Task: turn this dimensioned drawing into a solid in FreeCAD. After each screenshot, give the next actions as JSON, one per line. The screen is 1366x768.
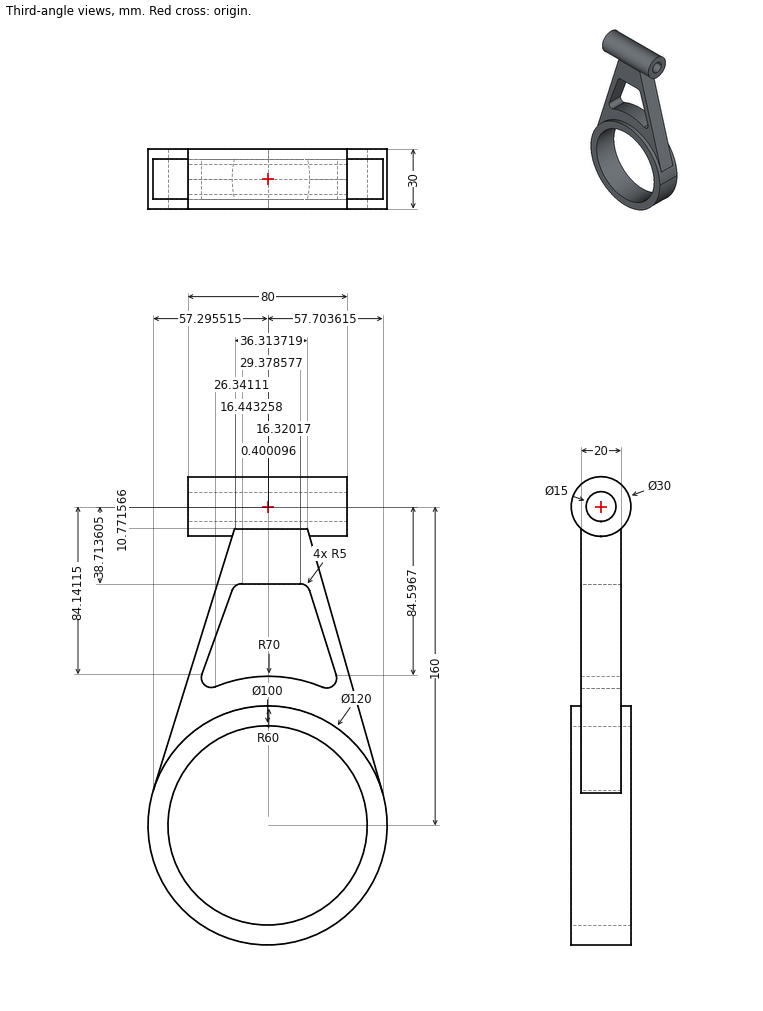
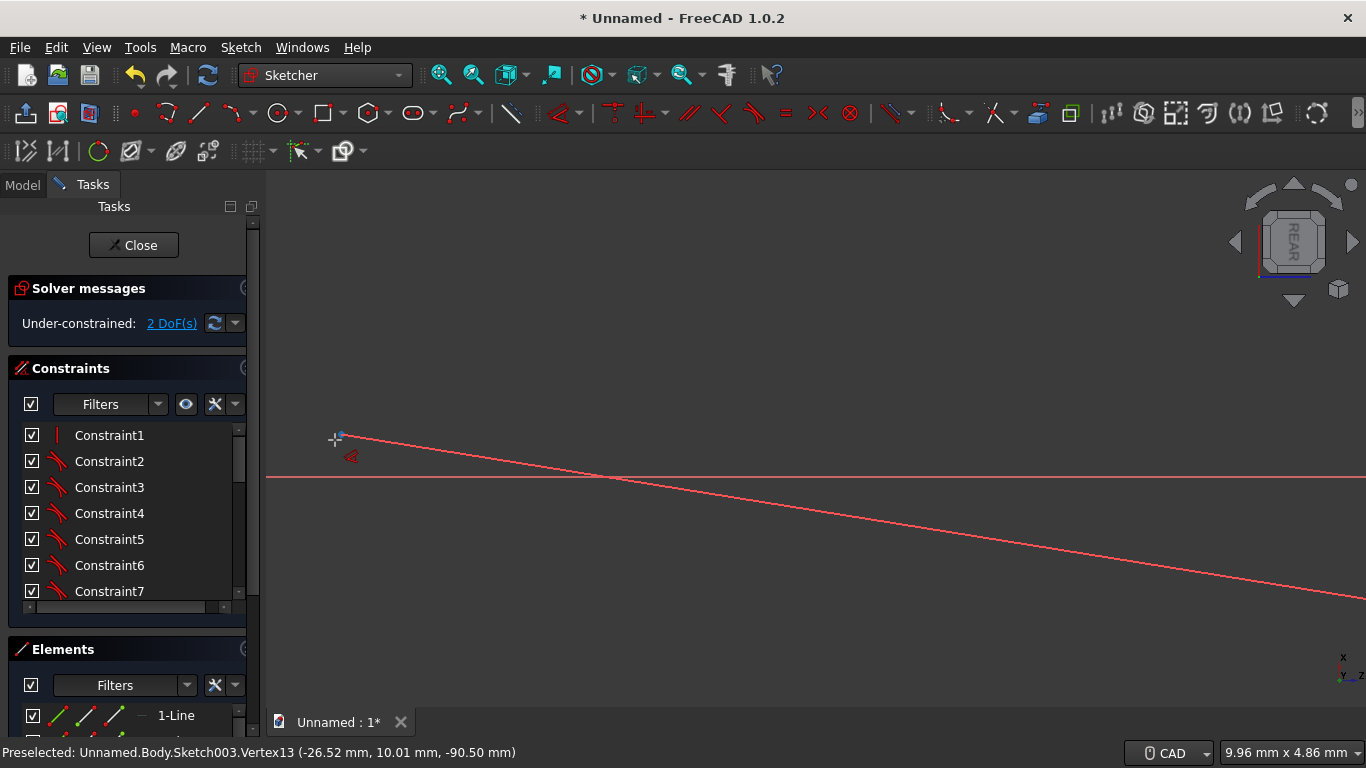
{"action": "left_click", "coordinate": [341, 435]}
{"action": "left_click", "coordinate": [307, 456]}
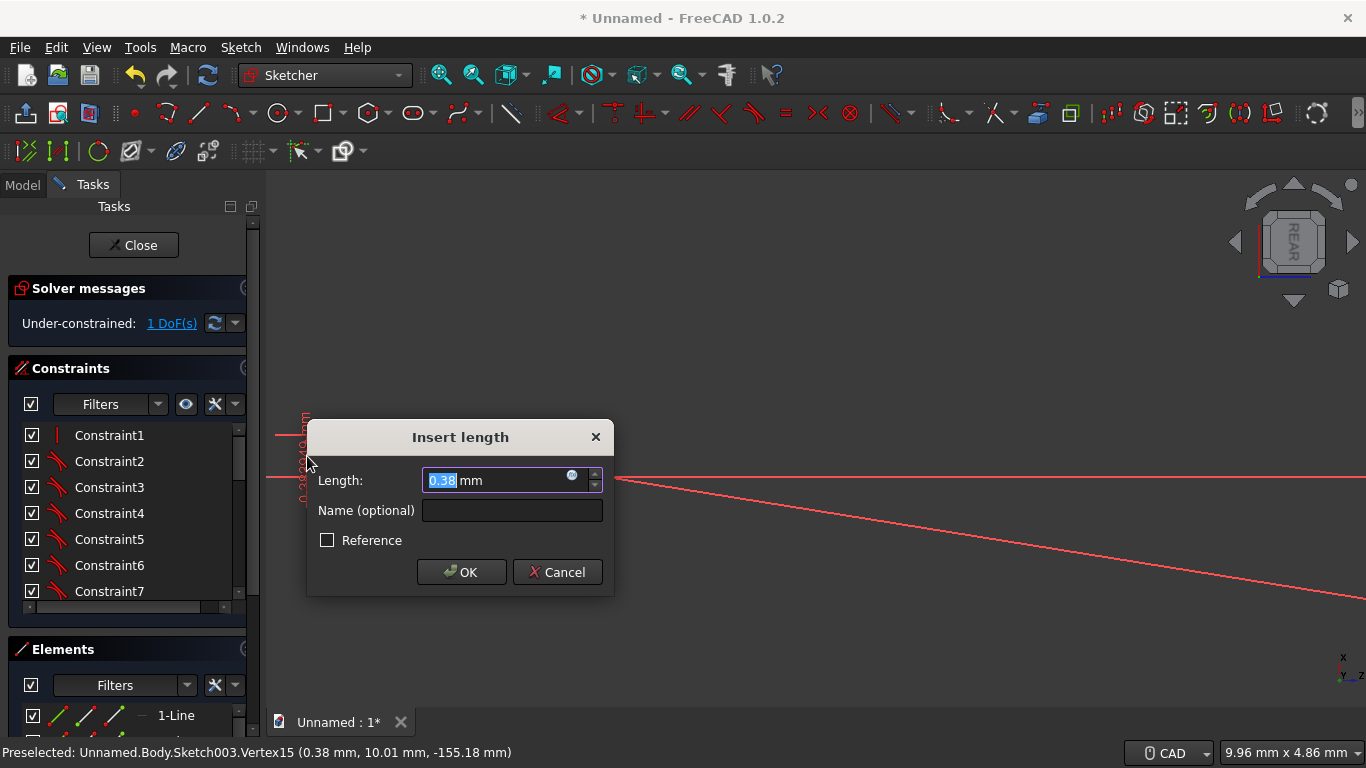
{"action": "type", "text": "0.400096"}
{"action": "key", "text": "Return"}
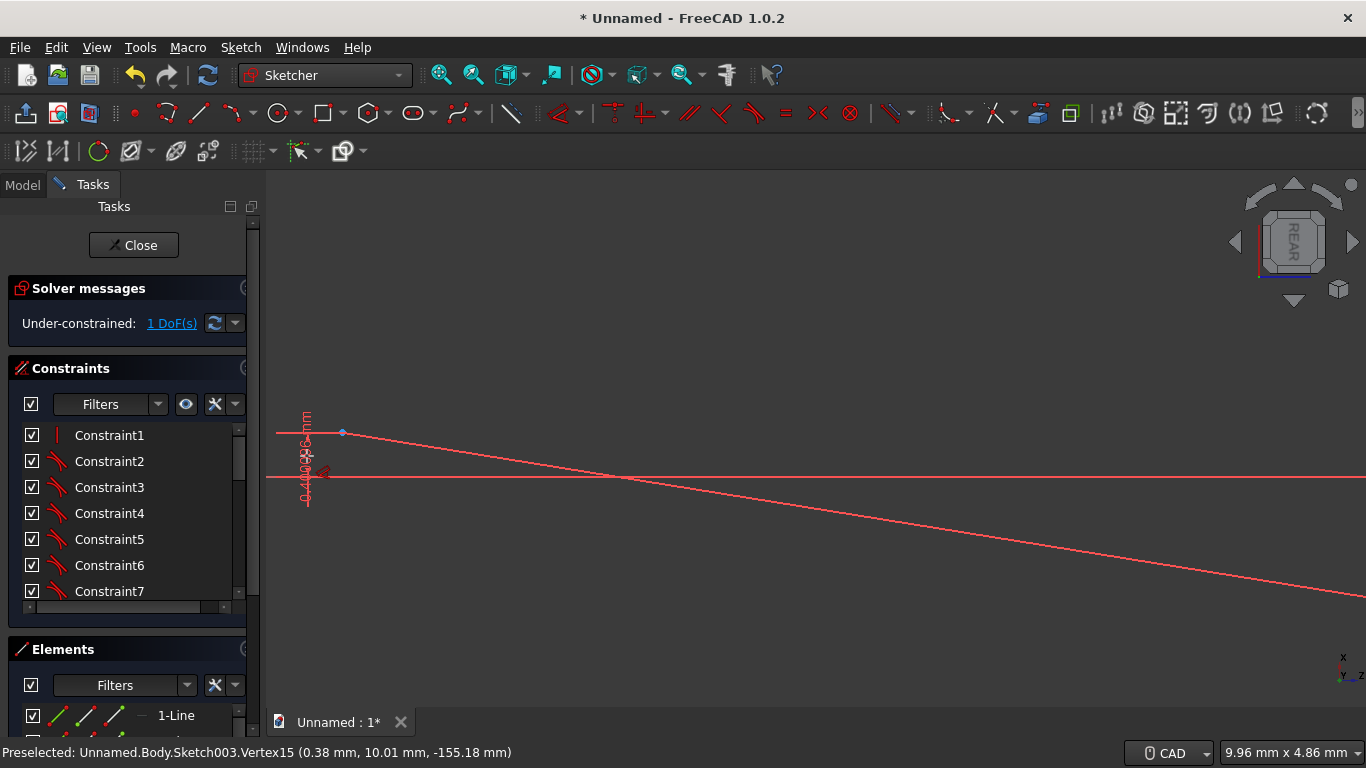
{"action": "scroll", "coordinate": [294, 441], "scroll_direction": "down", "scroll_amount": 15}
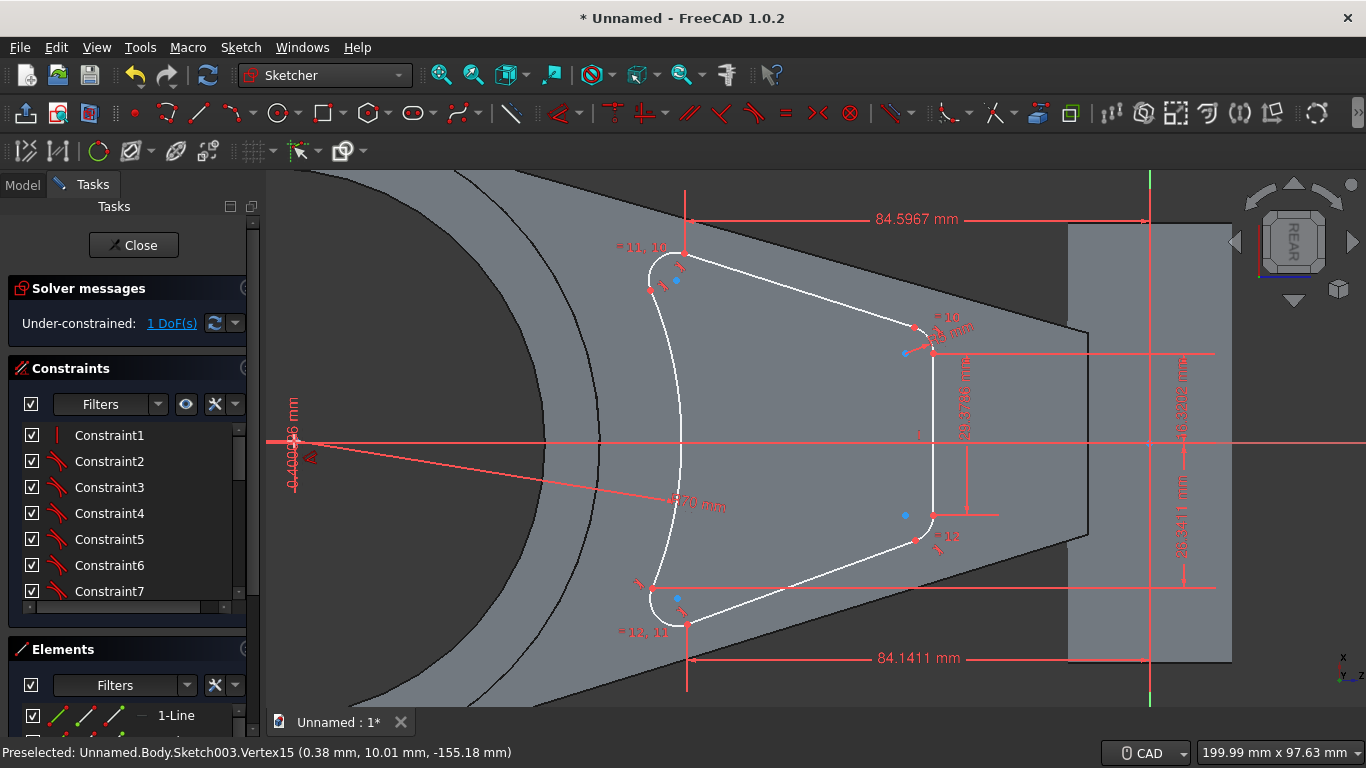
{"action": "left_click", "coordinate": [933, 515]}
{"action": "left_click", "coordinate": [1042, 549]}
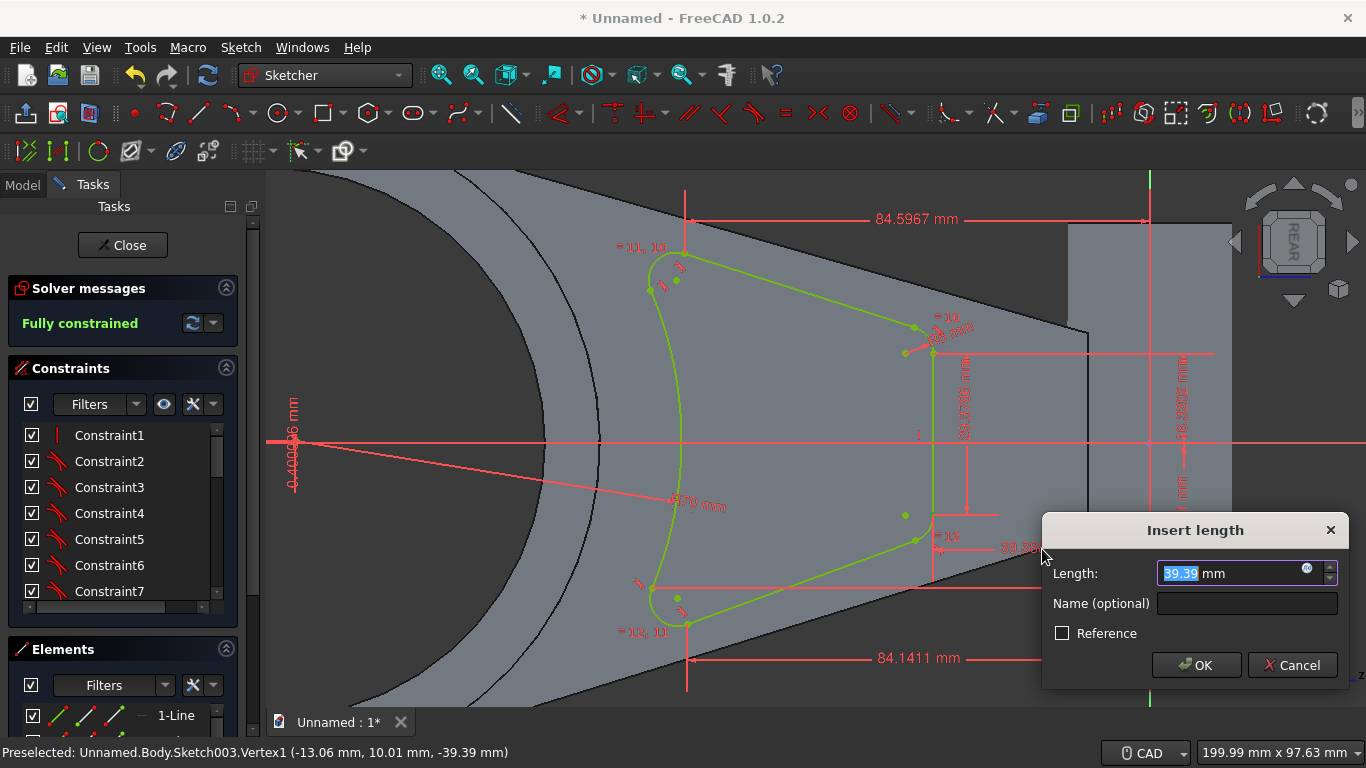
{"action": "type", "text": "38.713605"}
{"action": "key", "text": "Return"}
{"action": "key", "text": "Escape"}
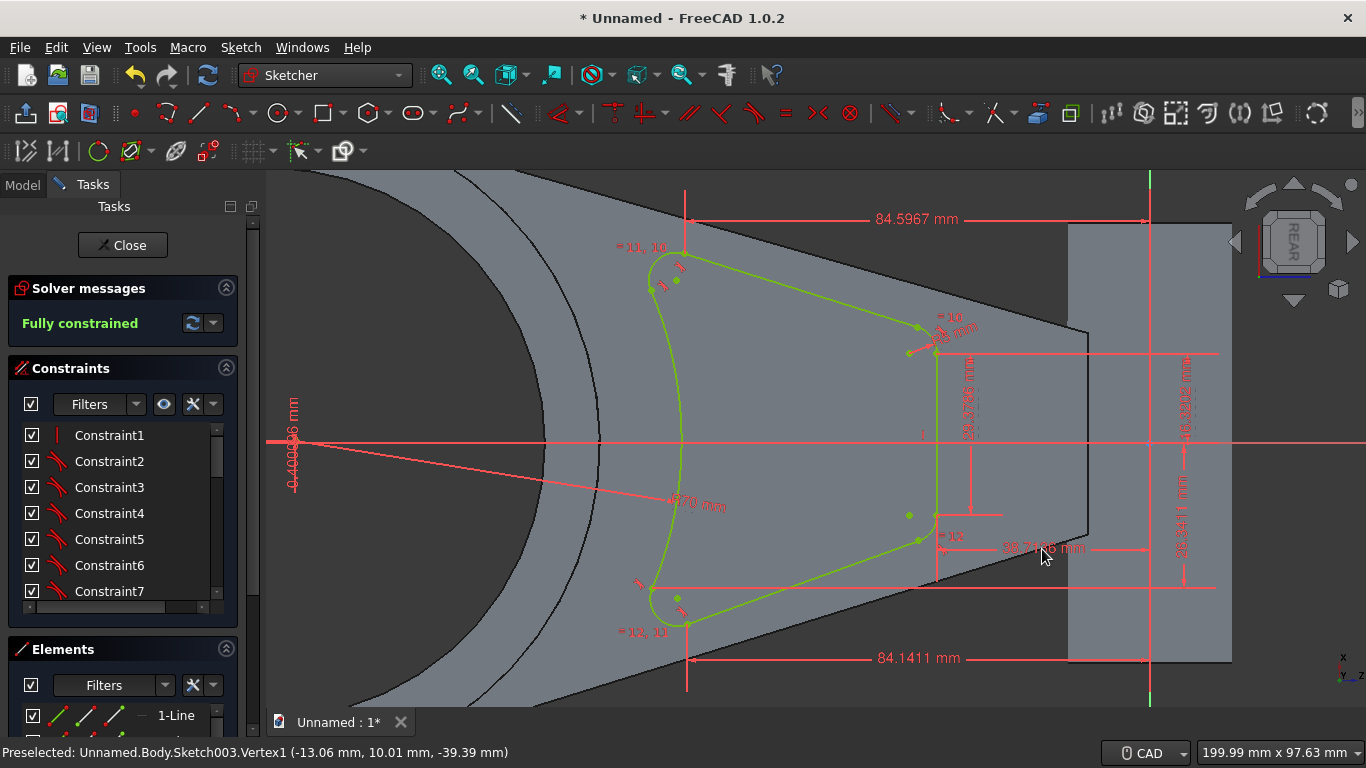
{"action": "left_click", "coordinate": [123, 245]}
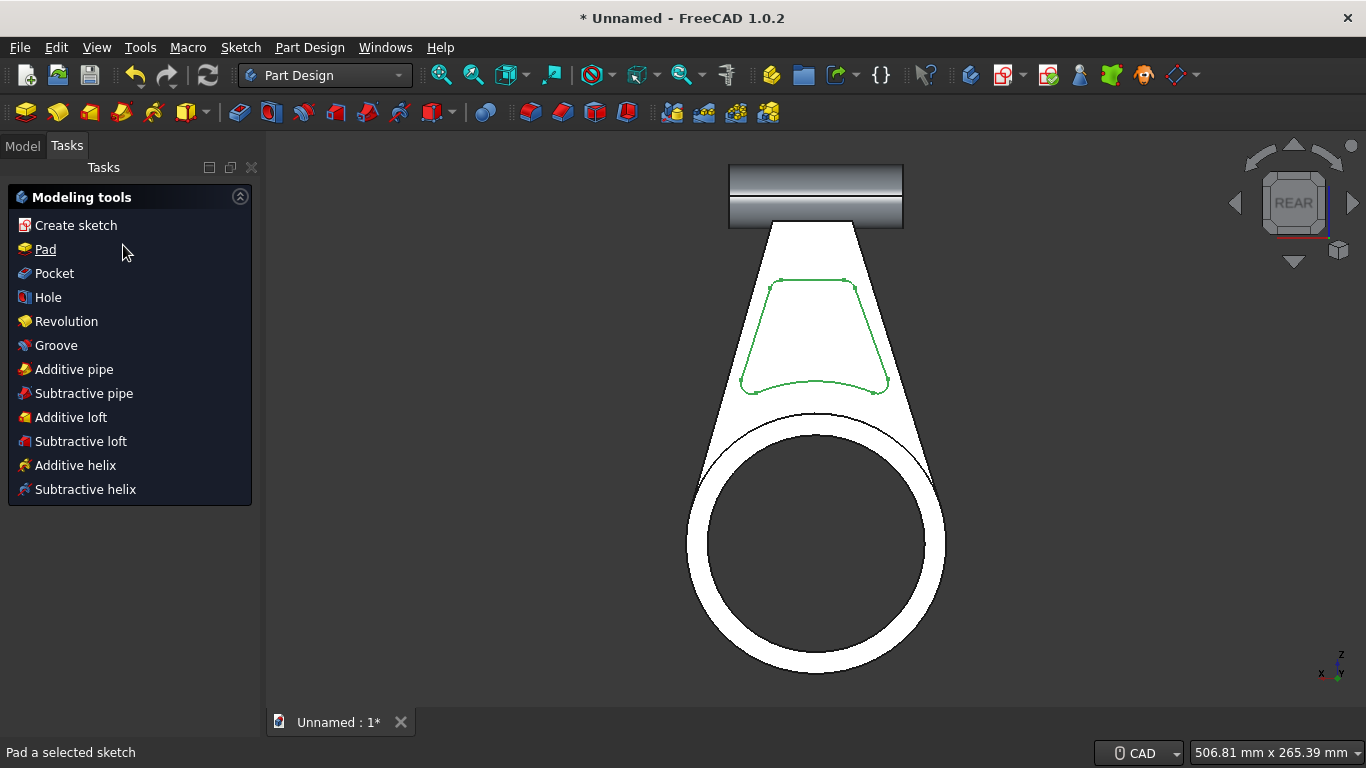
{"action": "left_click", "coordinate": [240, 112]}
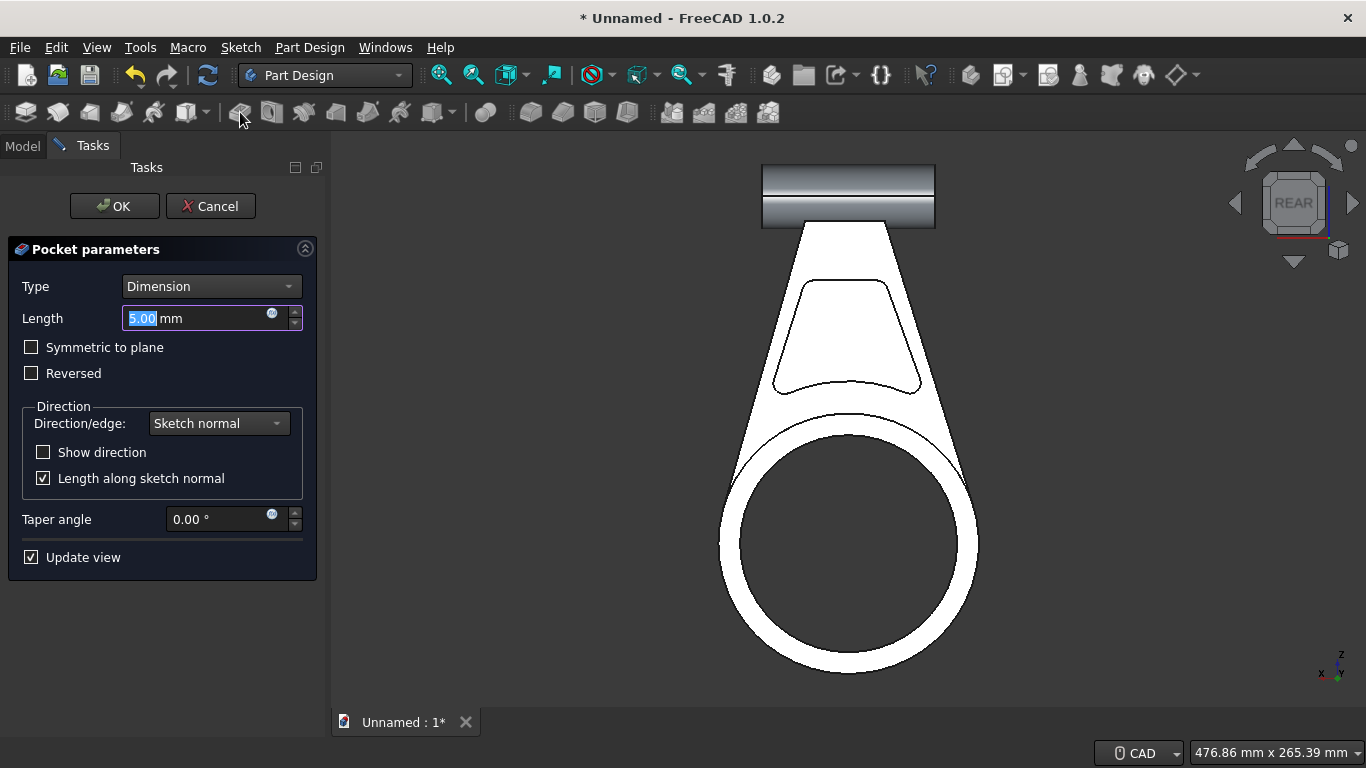
{"action": "left_click", "coordinate": [212, 286]}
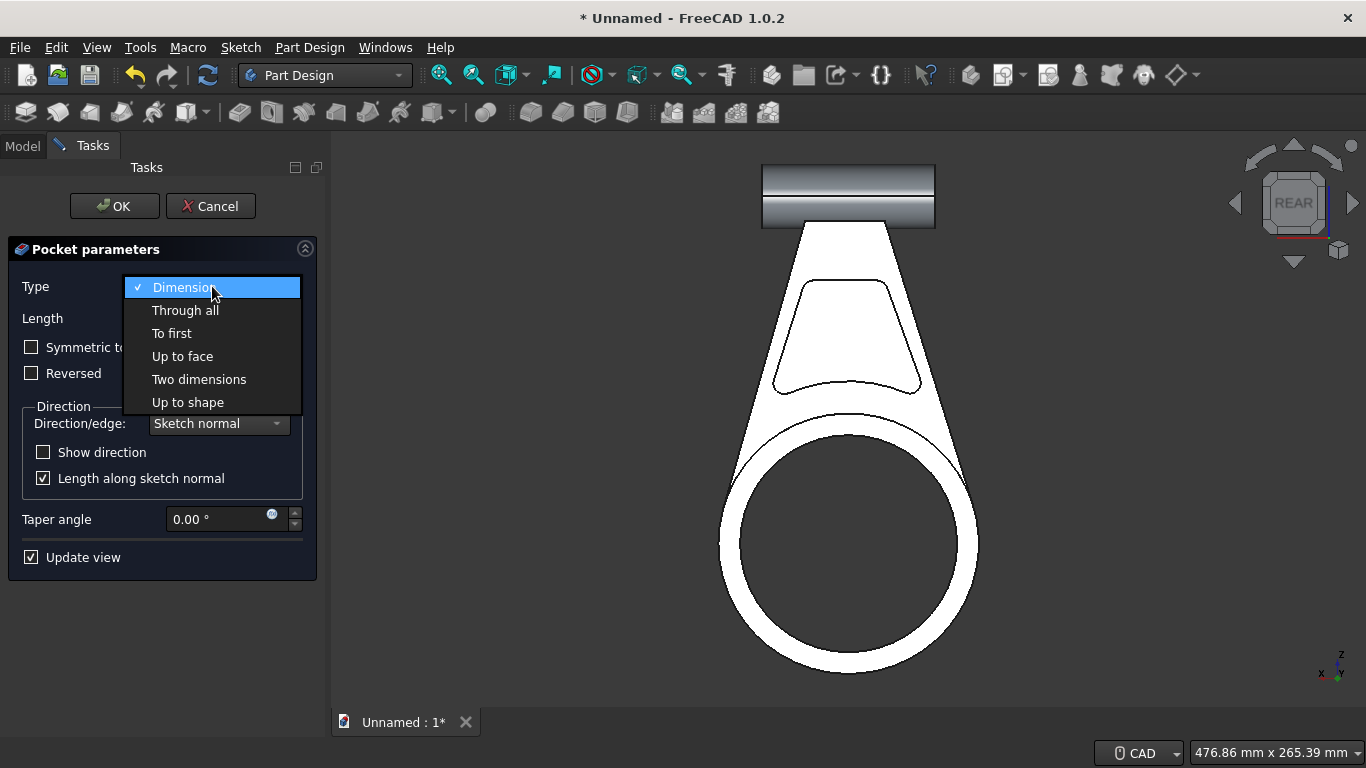
{"action": "left_click", "coordinate": [212, 310]}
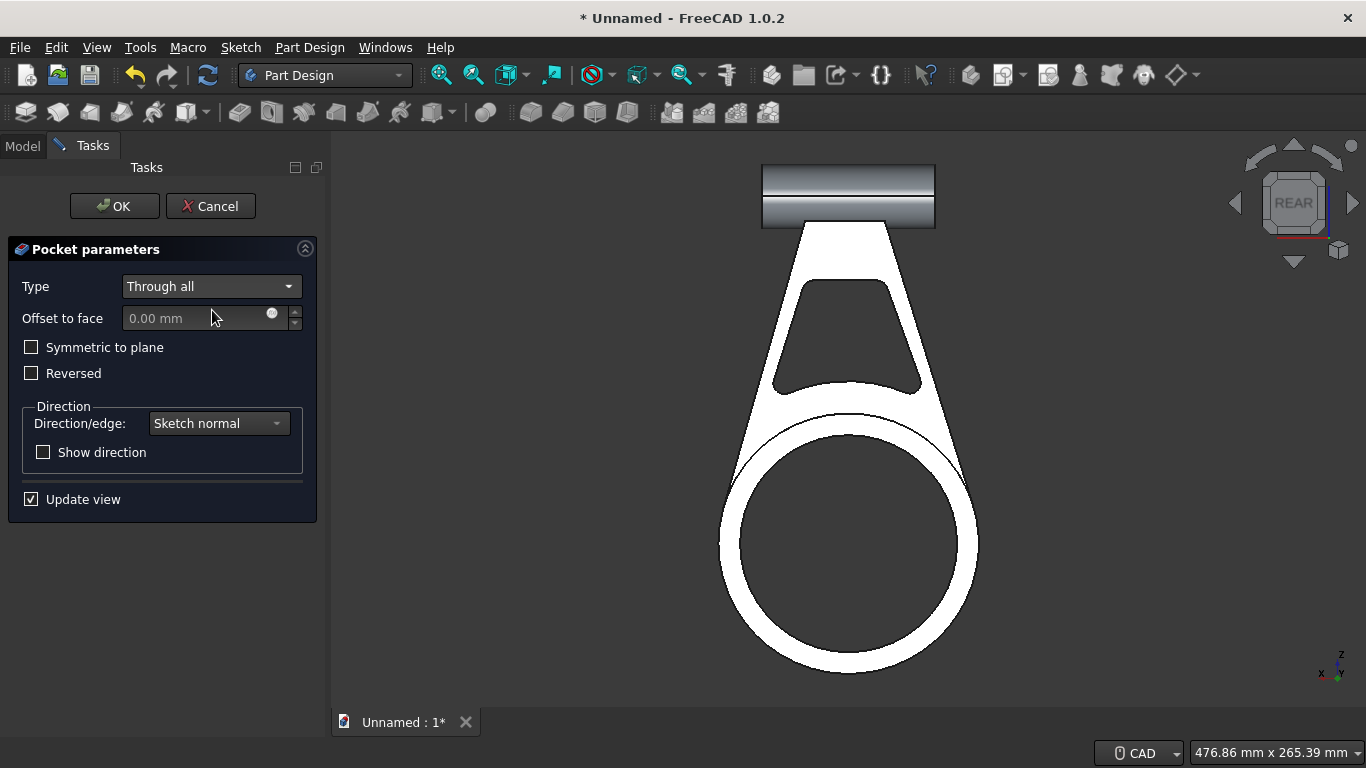
{"action": "left_click", "coordinate": [115, 206]}